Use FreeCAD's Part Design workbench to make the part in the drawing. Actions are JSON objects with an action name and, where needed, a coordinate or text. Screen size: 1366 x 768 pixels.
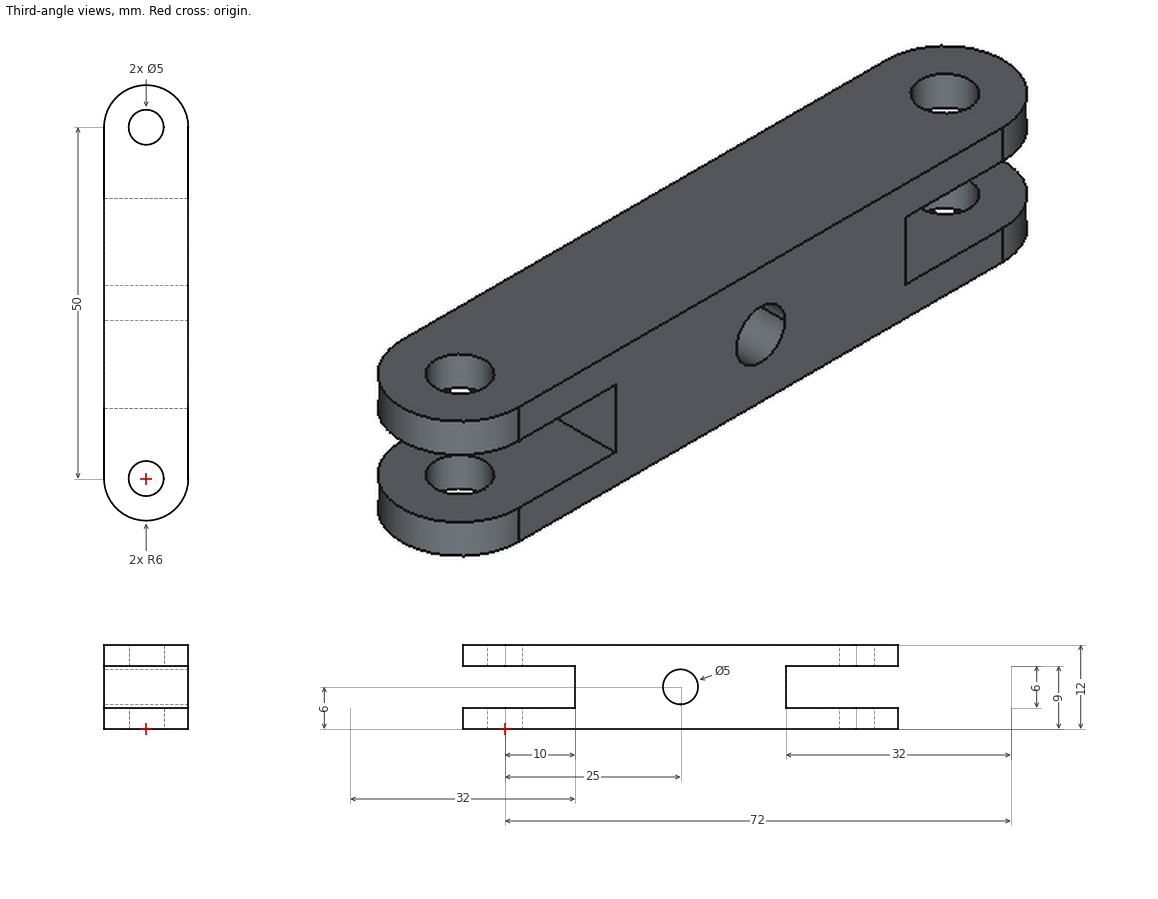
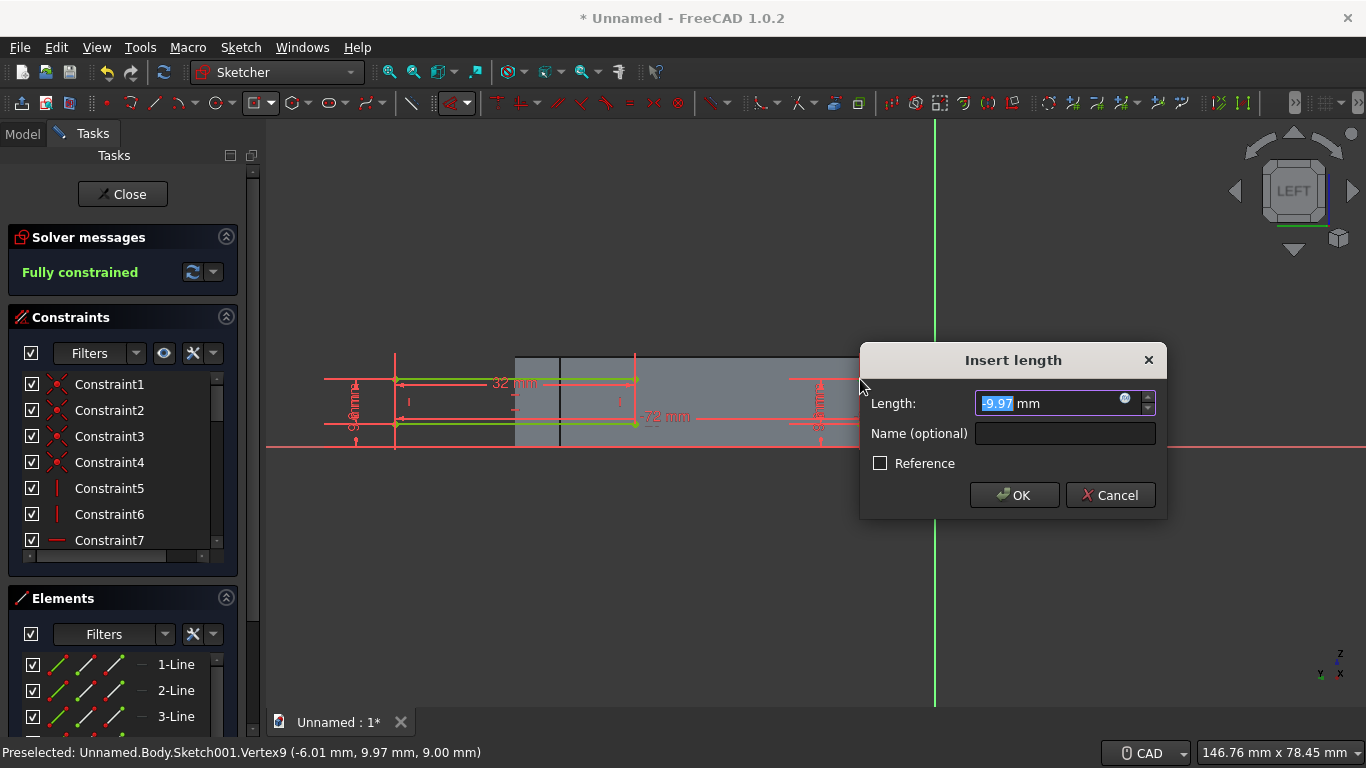
{"action": "type", "text": "-10"}
{"action": "key", "text": "Return"}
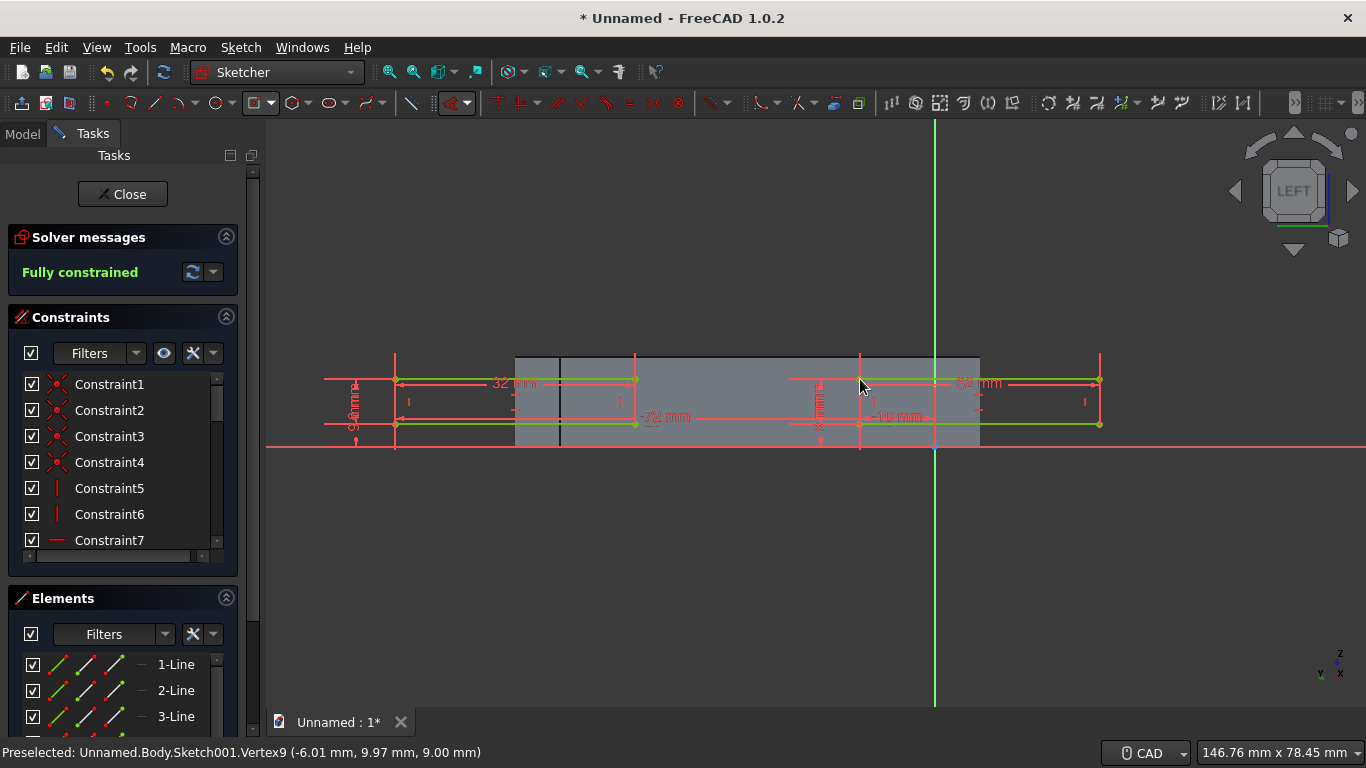
{"action": "left_click", "coordinate": [123, 194]}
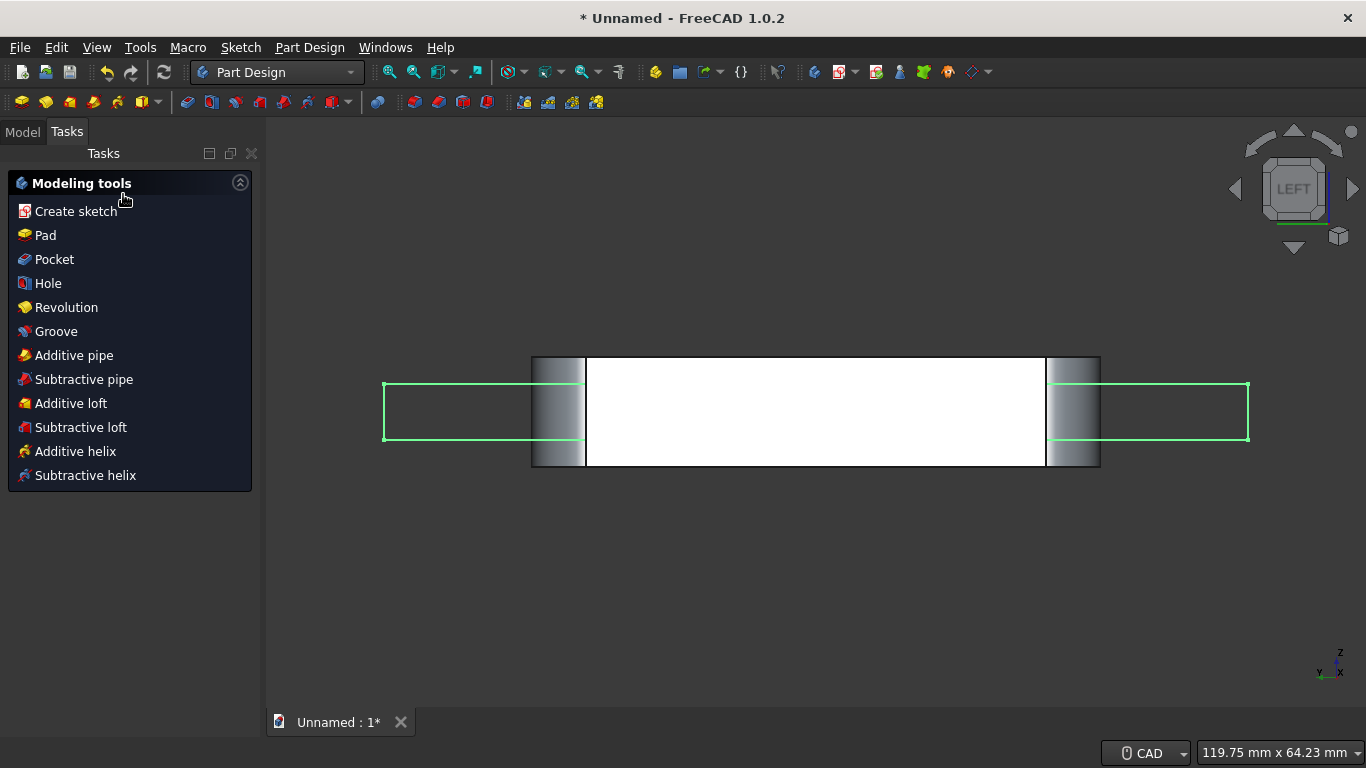
{"action": "left_click", "coordinate": [188, 102]}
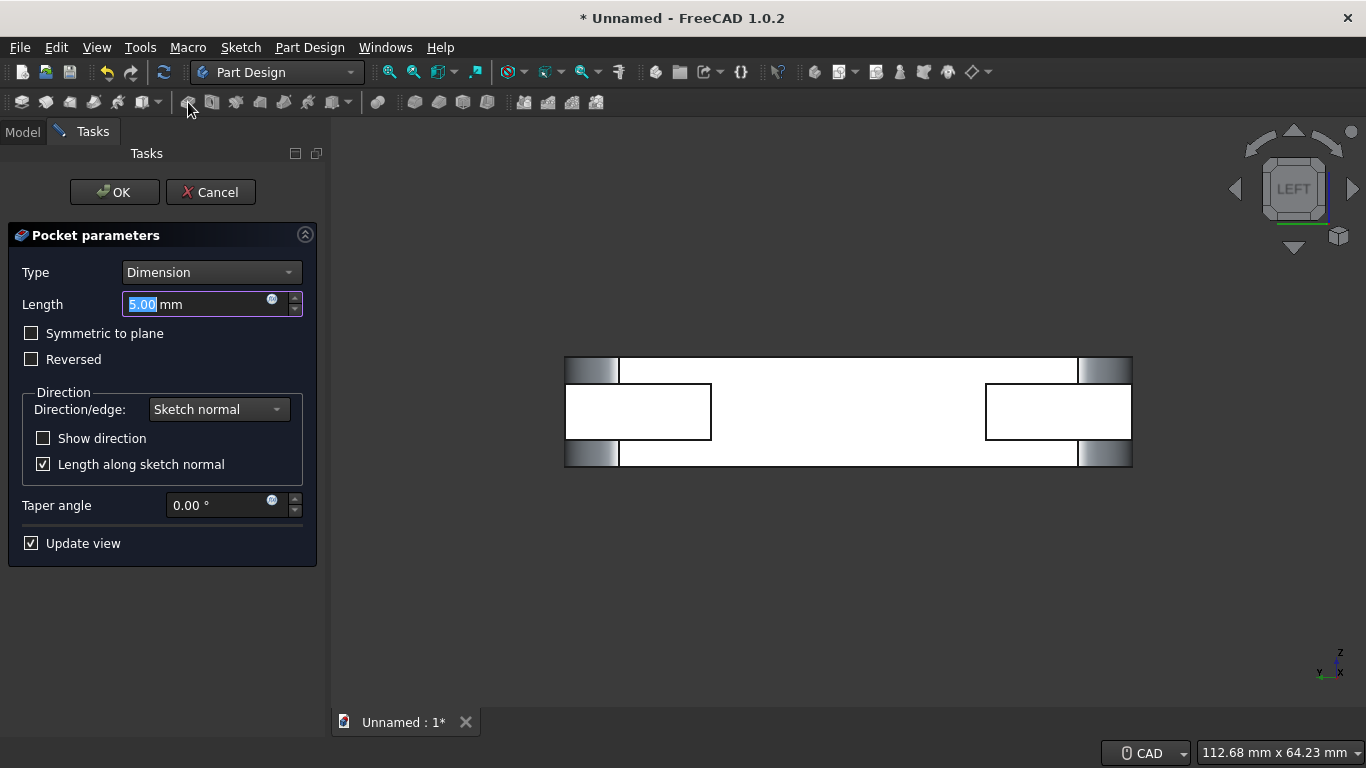
{"action": "left_click", "coordinate": [212, 272]}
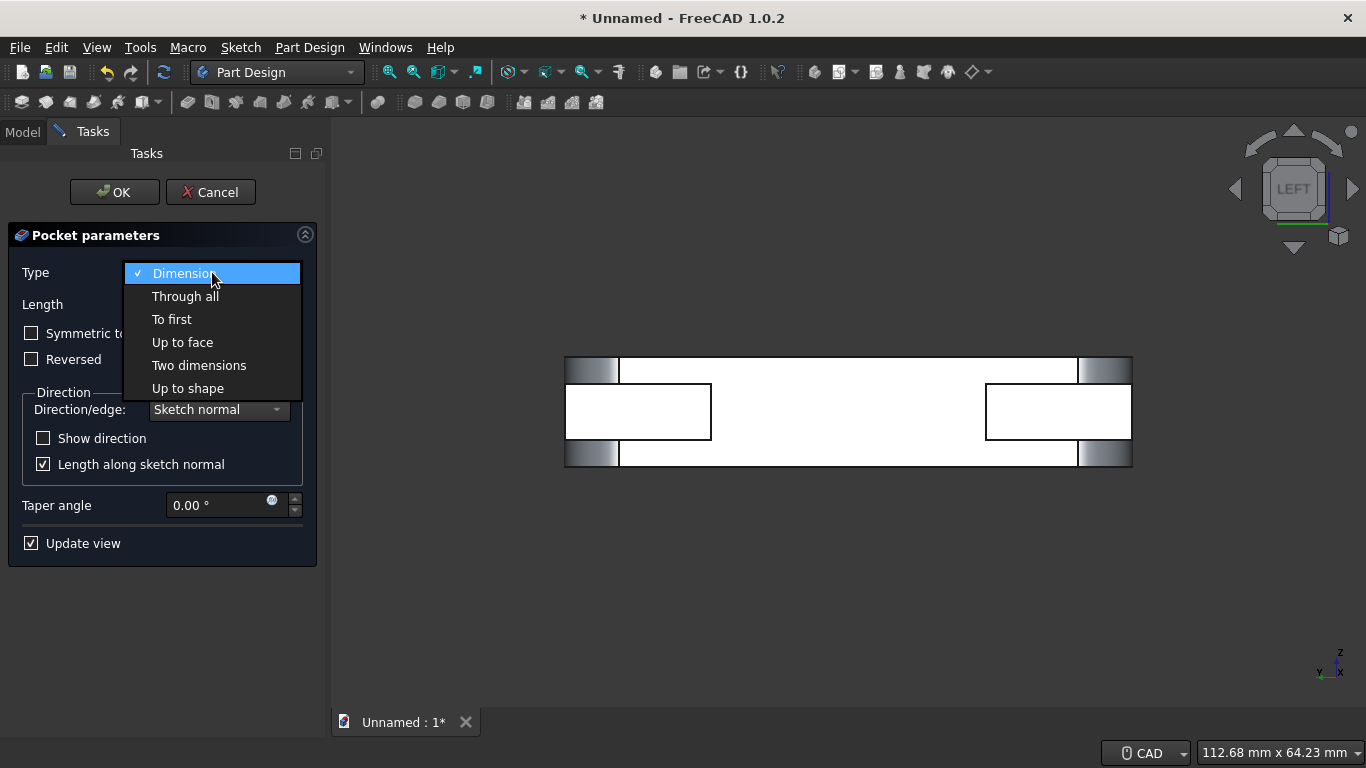
{"action": "left_click", "coordinate": [212, 296]}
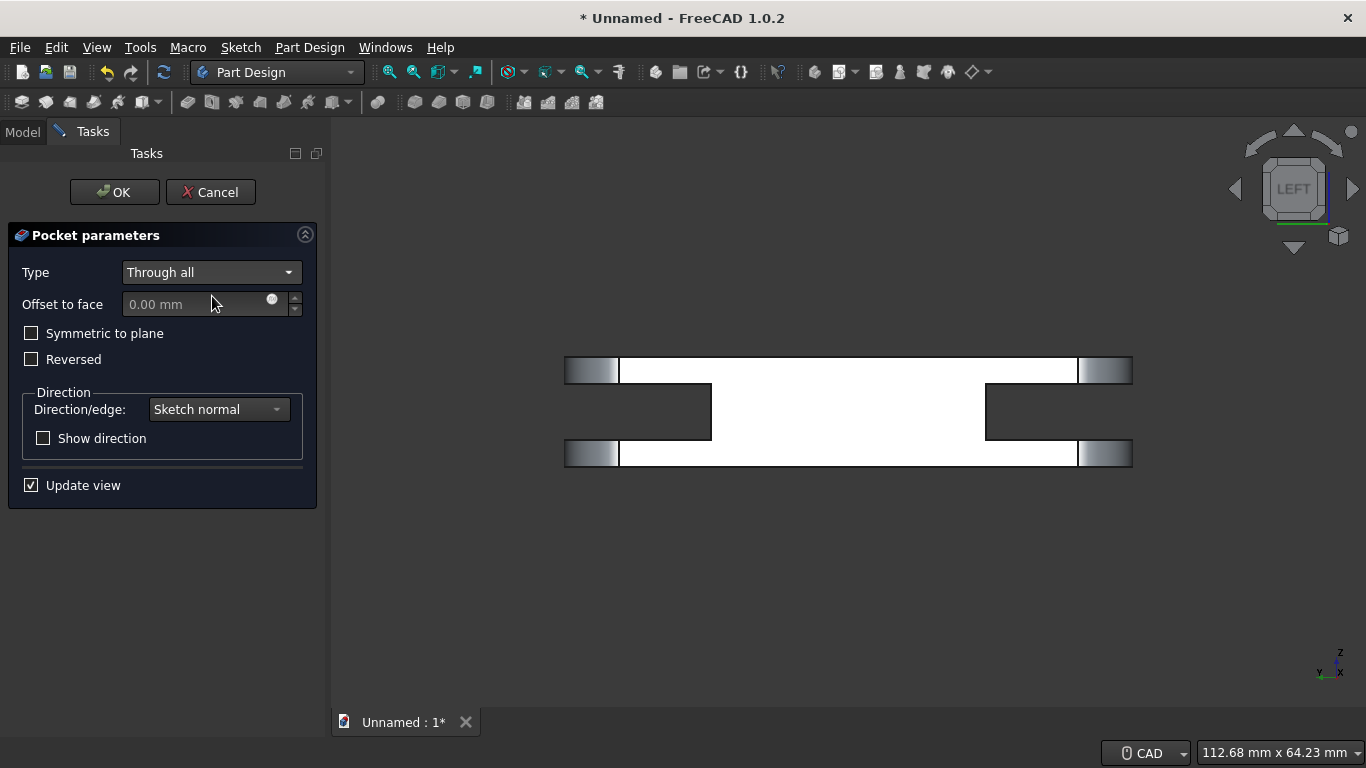
{"action": "left_click", "coordinate": [115, 192]}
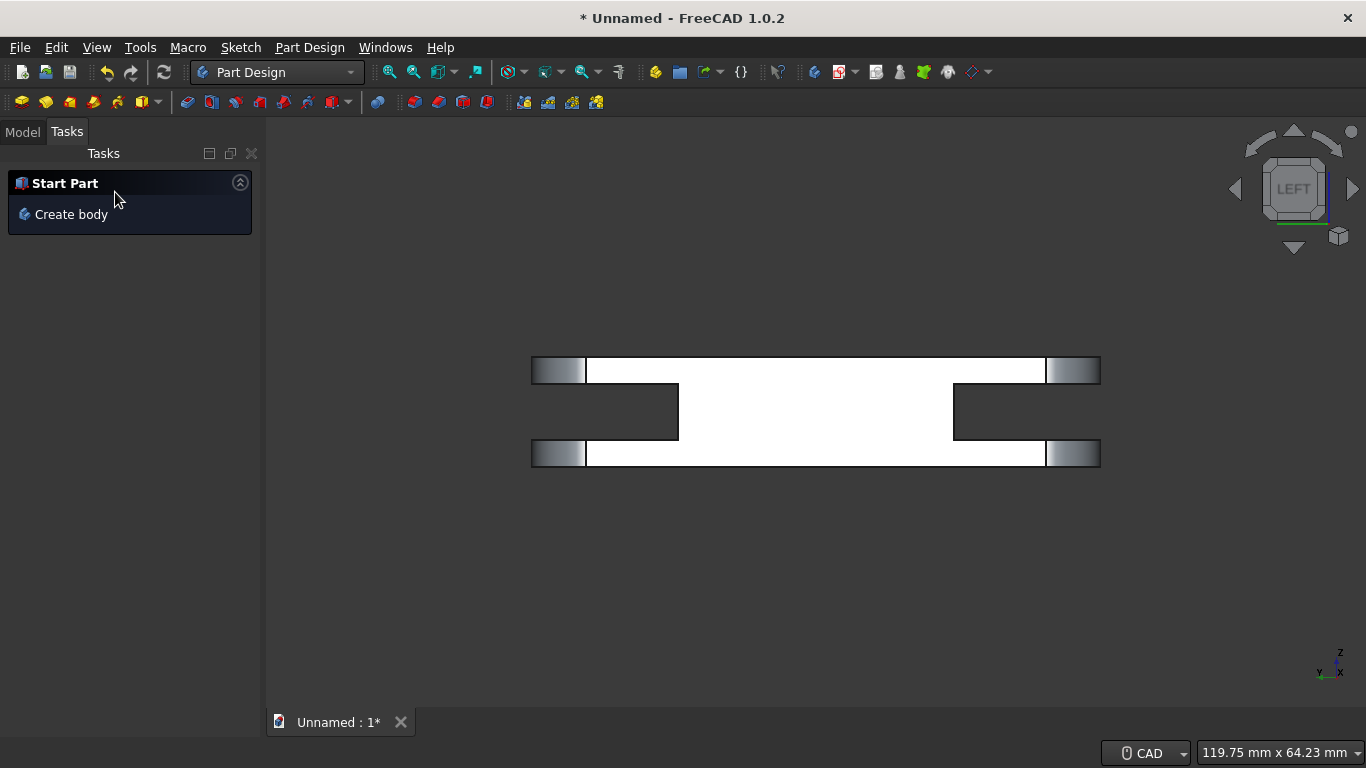
{"action": "key", "text": "0"}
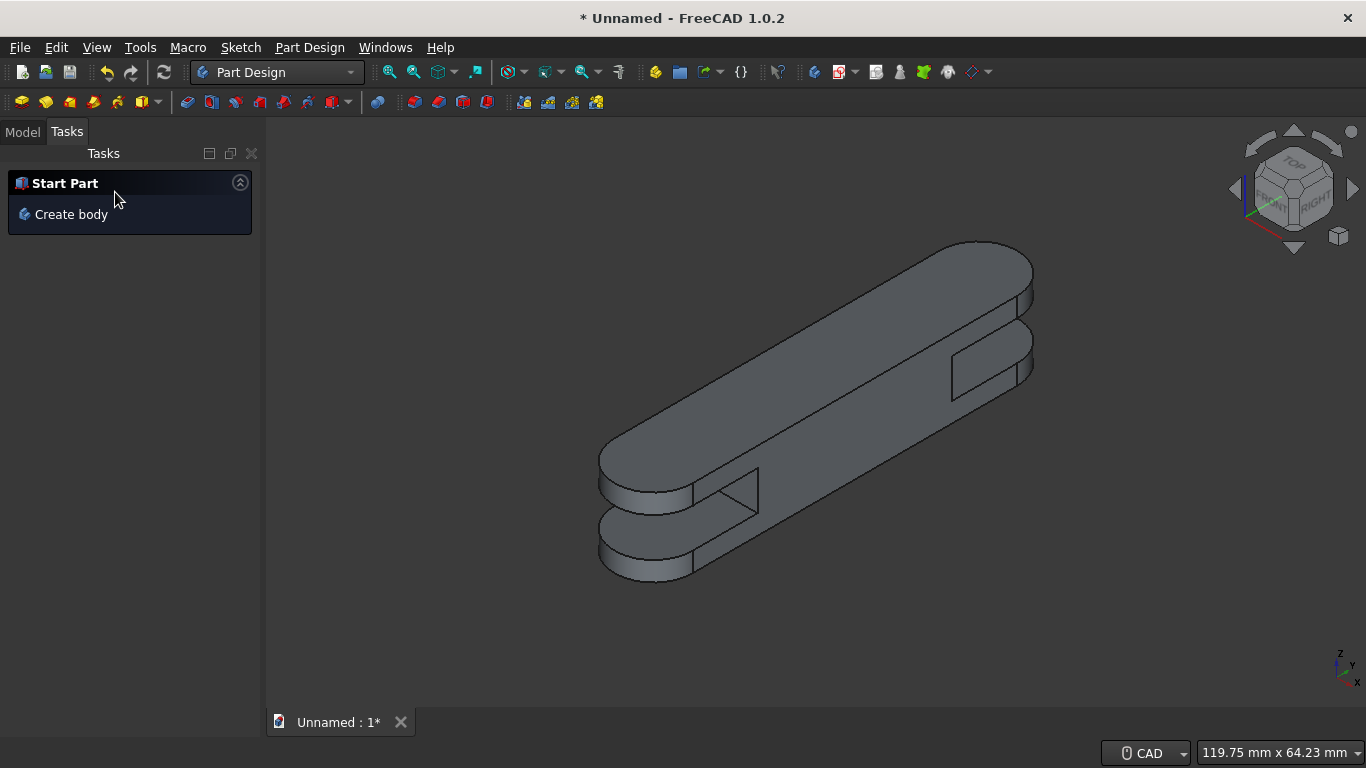
{"action": "left_click", "coordinate": [931, 300]}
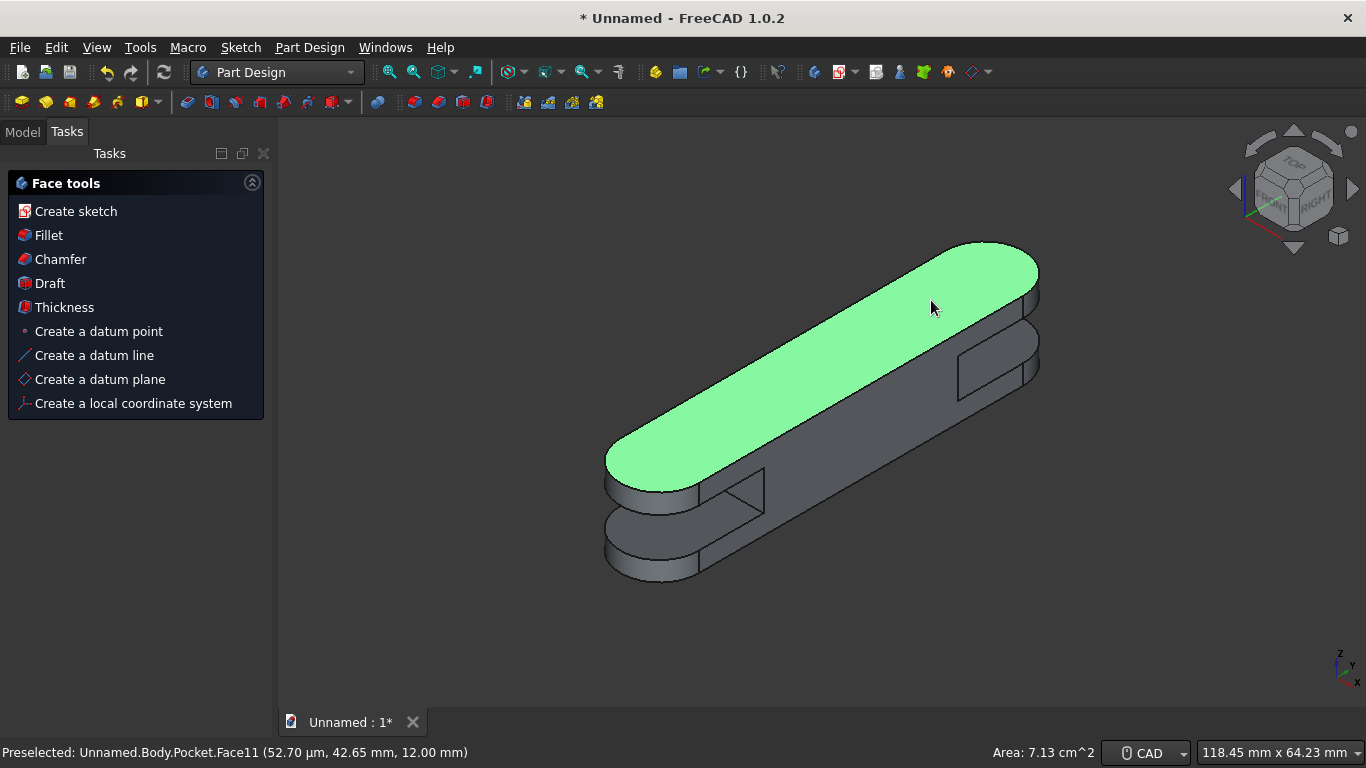
{"action": "left_click", "coordinate": [840, 72]}